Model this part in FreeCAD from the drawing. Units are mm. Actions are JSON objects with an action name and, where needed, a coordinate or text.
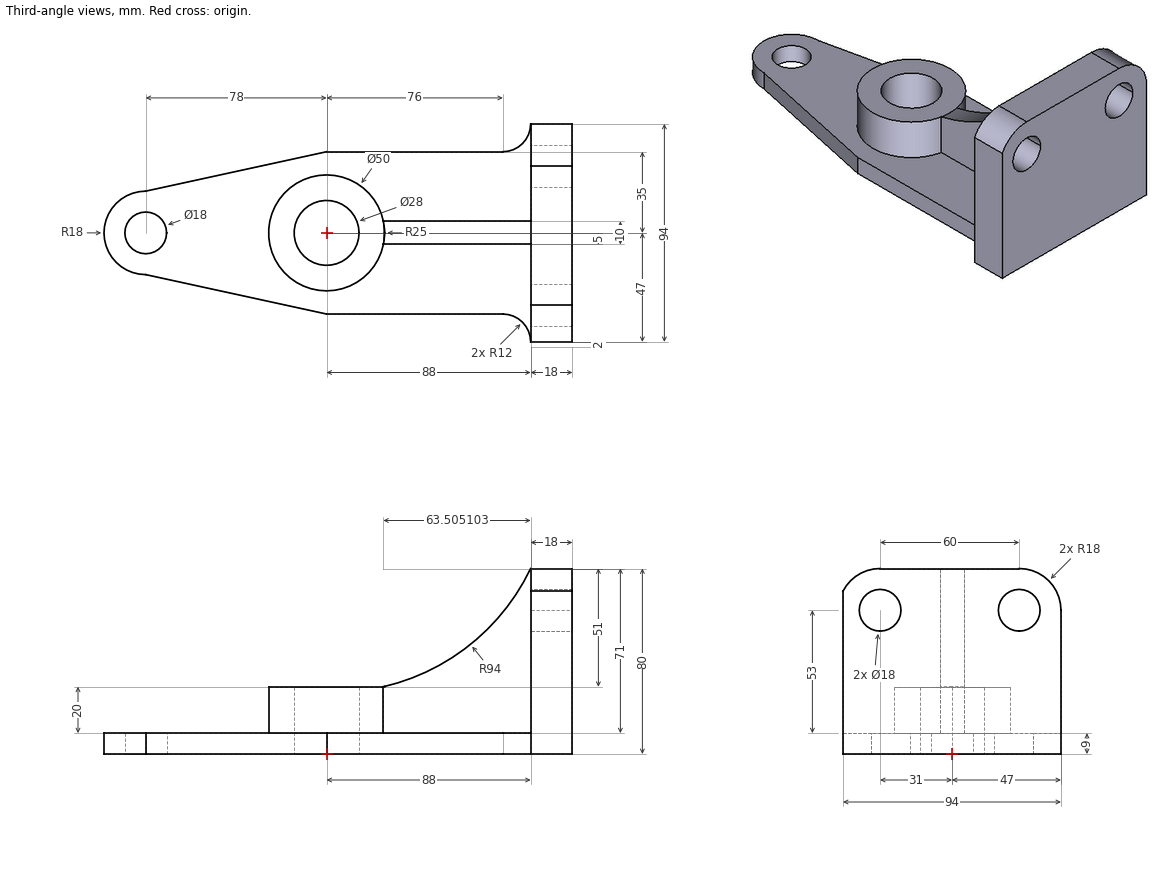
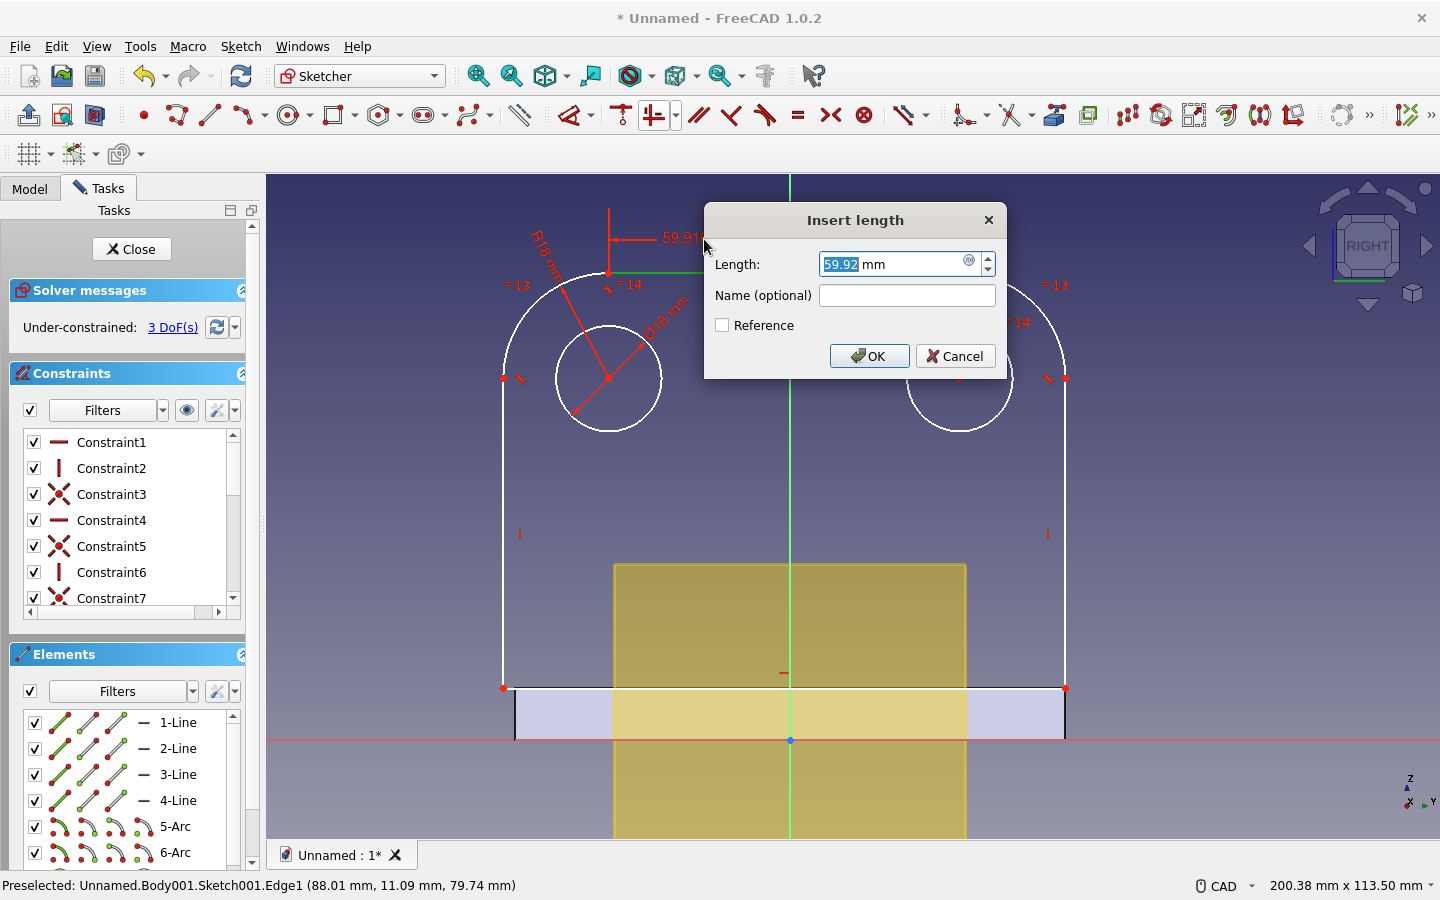
{"action": "type", "text": "60"}
{"action": "key", "text": "Return"}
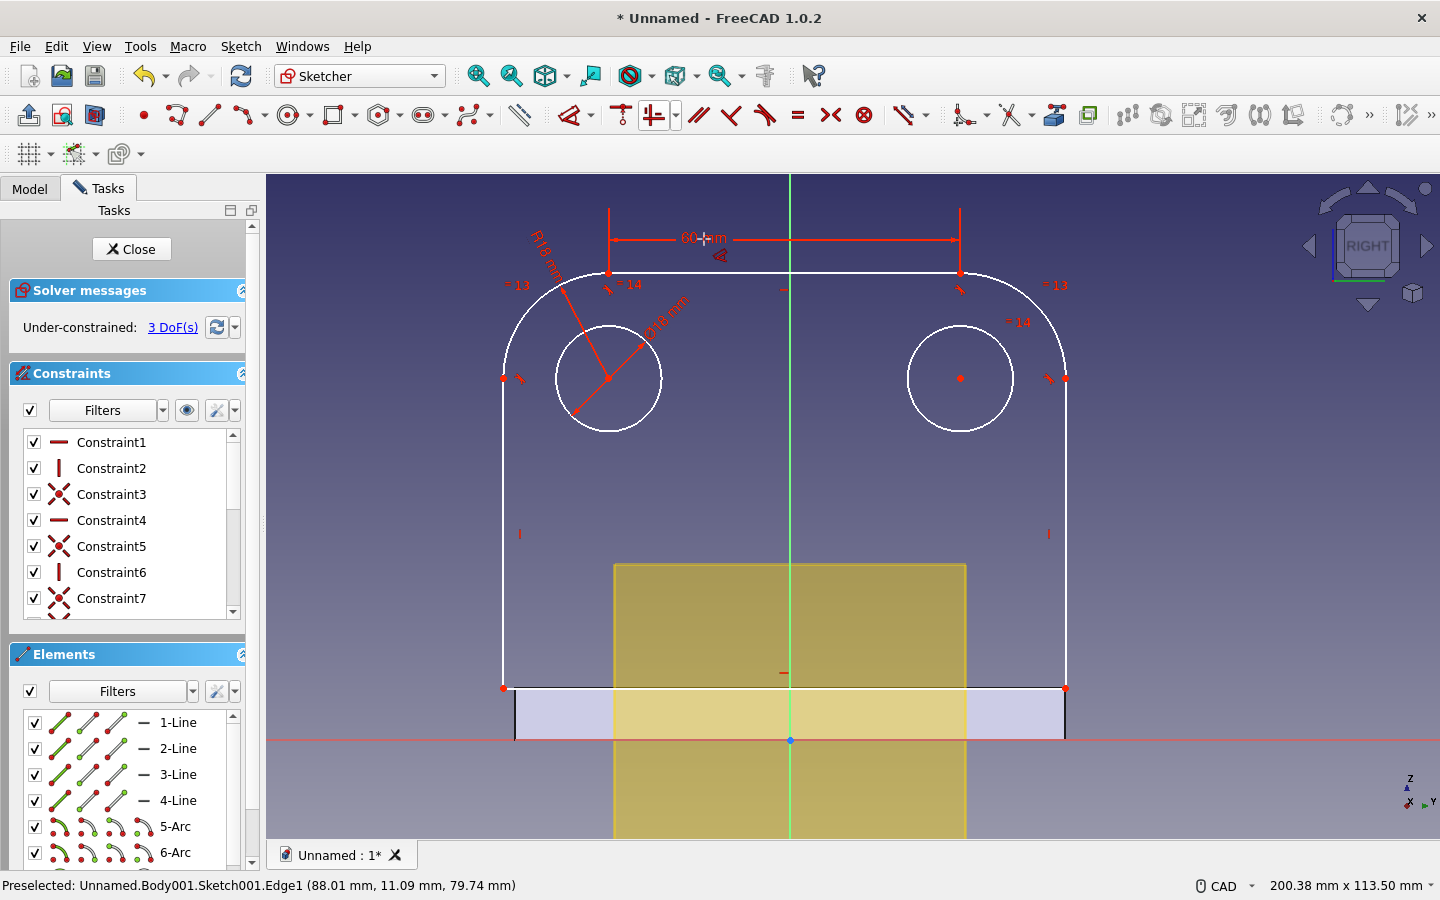
{"action": "left_click", "coordinate": [503, 472]}
{"action": "left_click", "coordinate": [469, 534]}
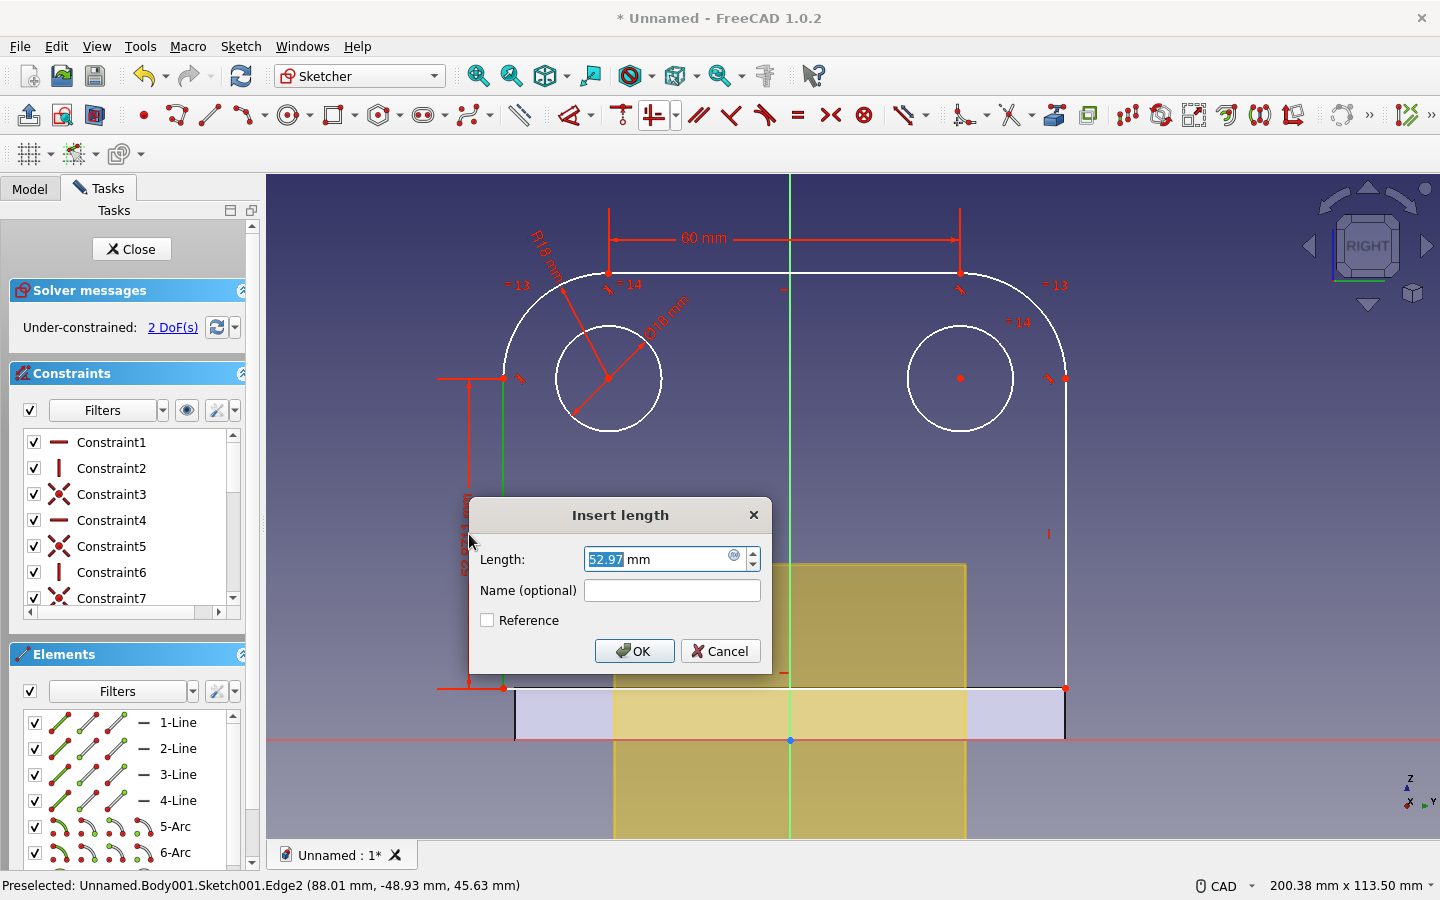
{"action": "type", "text": "53"}
{"action": "key", "text": "Return"}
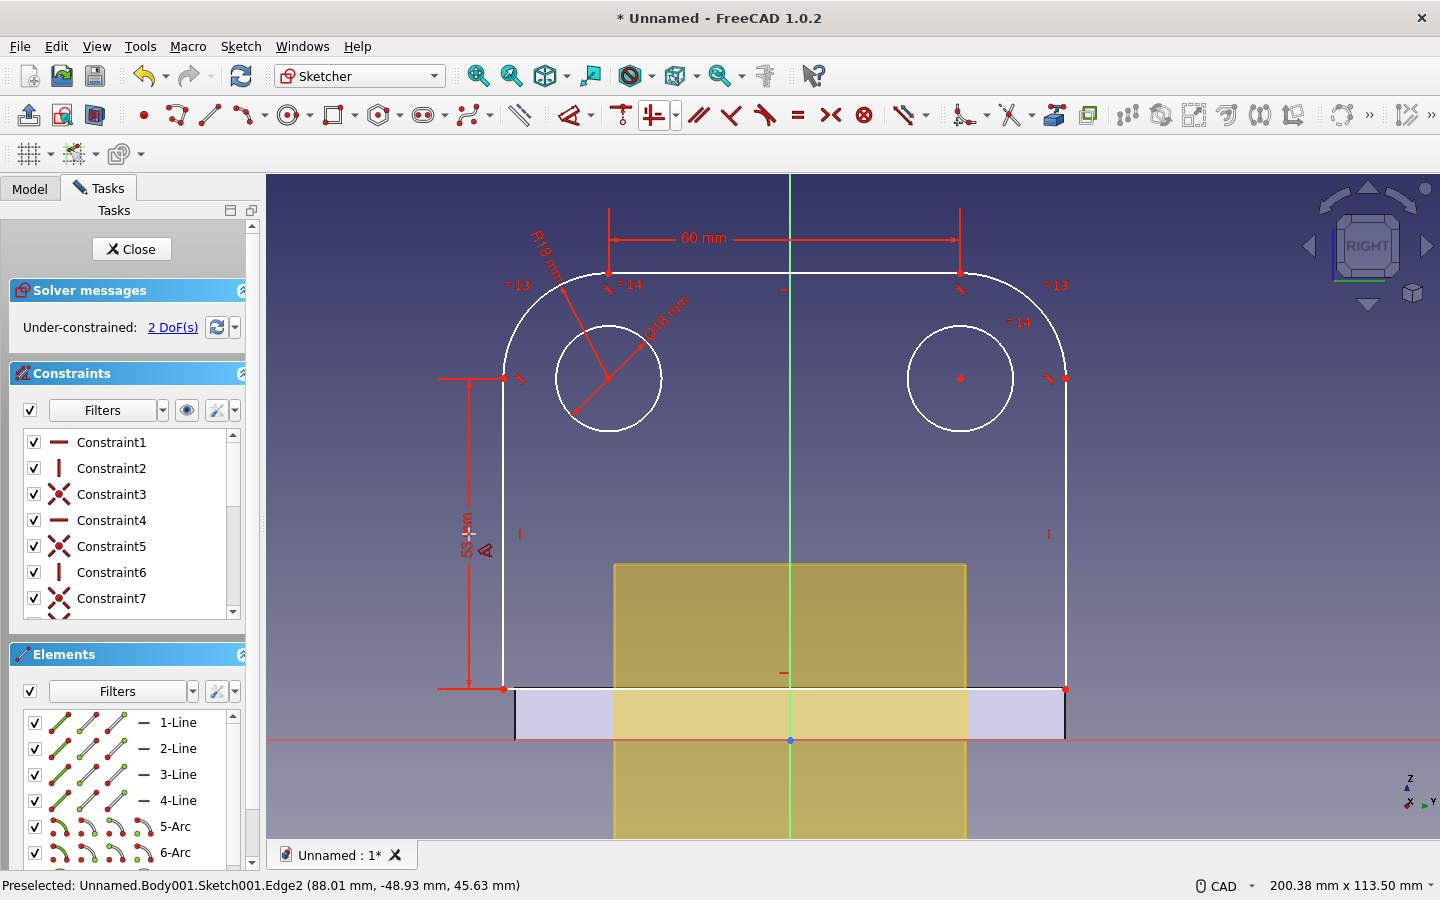
{"action": "left_click", "coordinate": [503, 689]}
{"action": "left_click", "coordinate": [469, 715]}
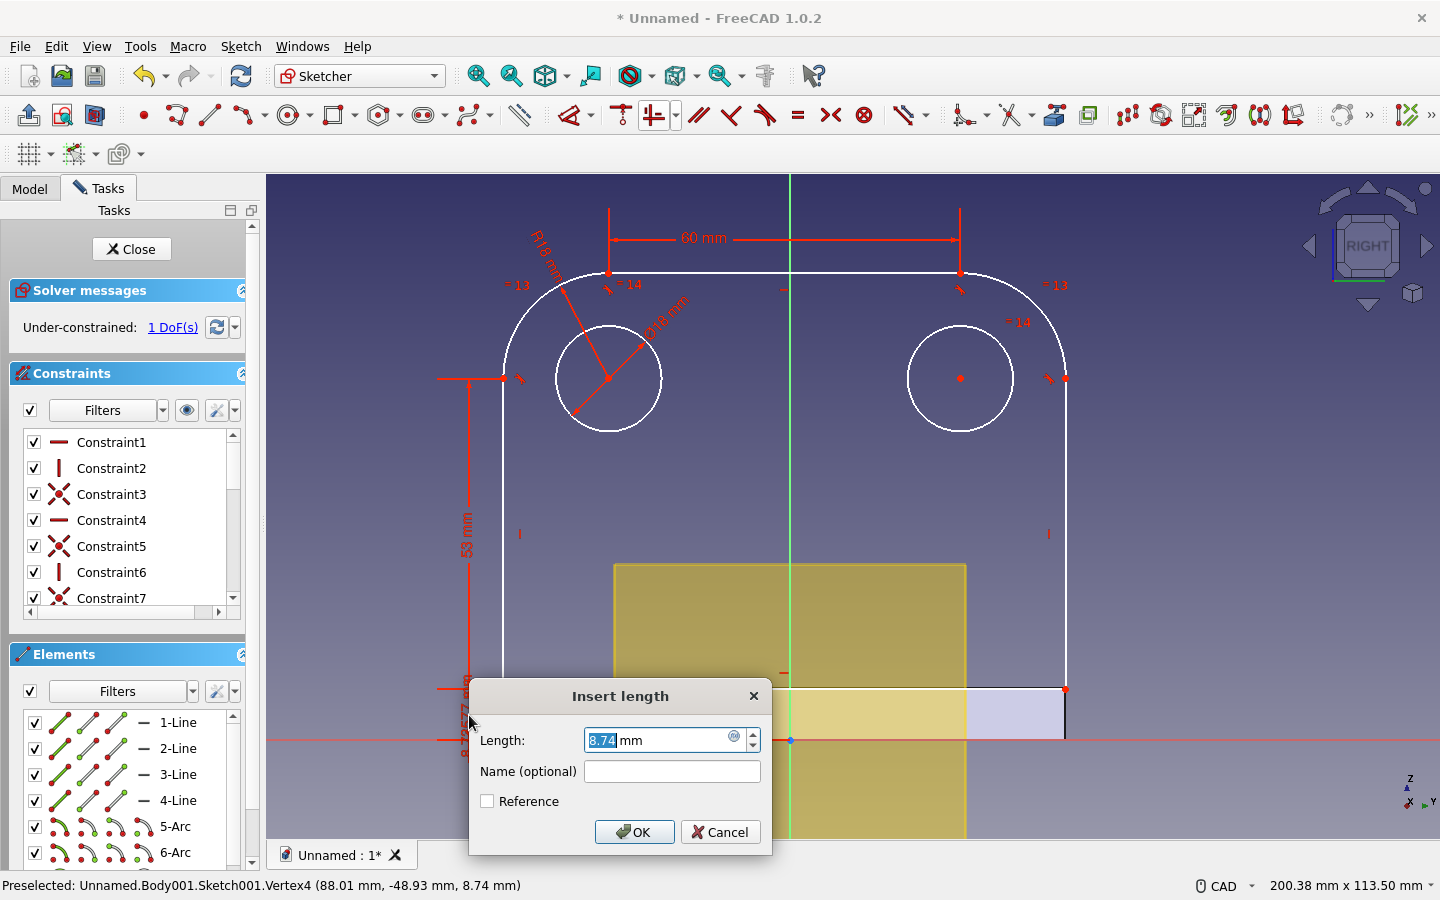
{"action": "type", "text": "9"}
{"action": "key", "text": "Return"}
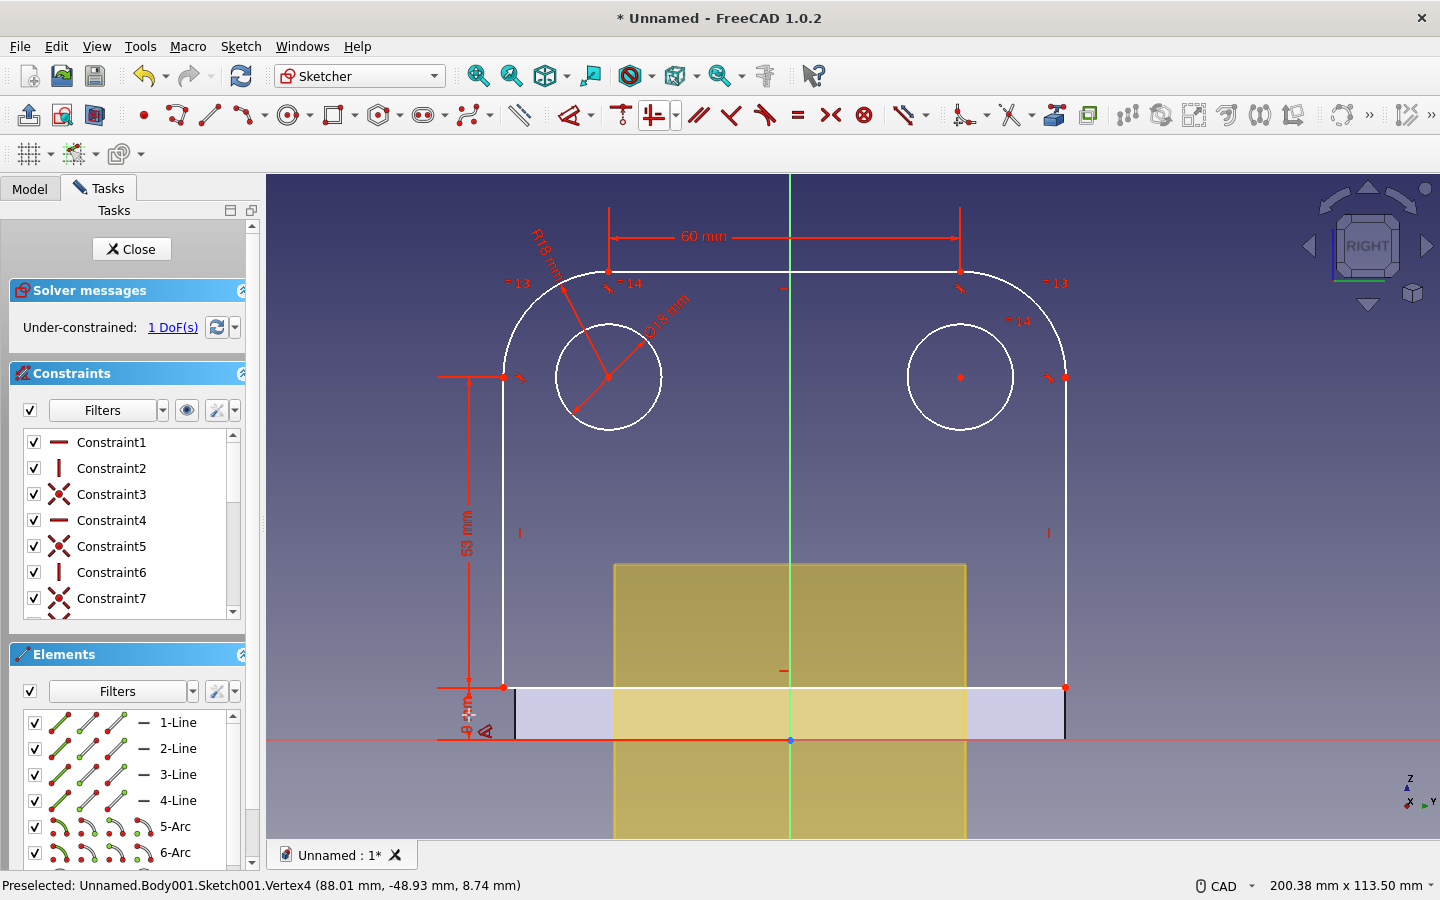
{"action": "left_click", "coordinate": [609, 377]}
{"action": "left_click", "coordinate": [699, 774]}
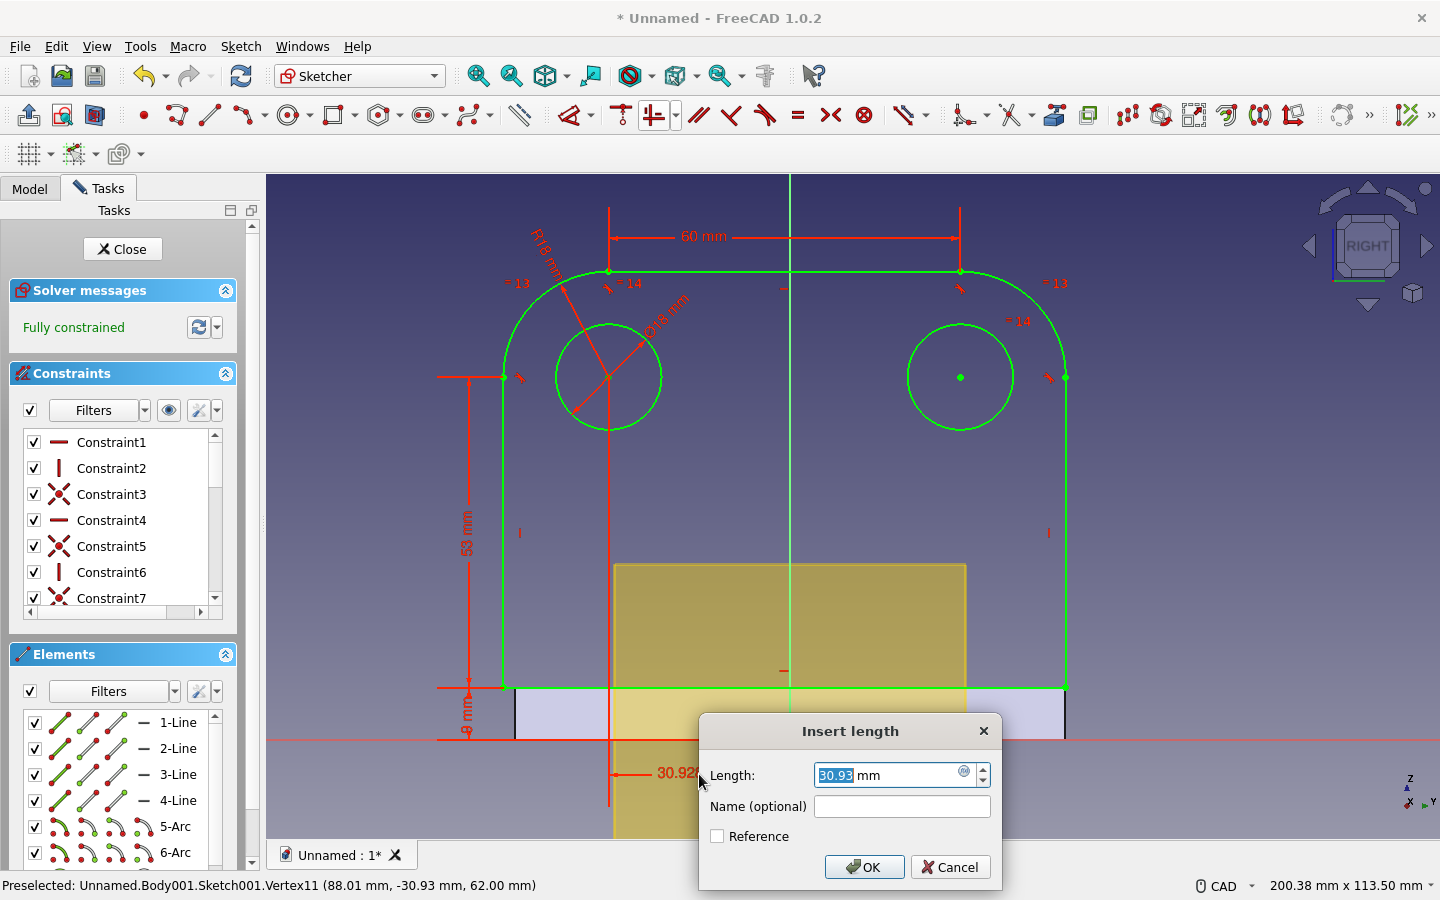
{"action": "type", "text": "31"}
{"action": "key", "text": "Return"}
{"action": "key", "text": "Escape"}